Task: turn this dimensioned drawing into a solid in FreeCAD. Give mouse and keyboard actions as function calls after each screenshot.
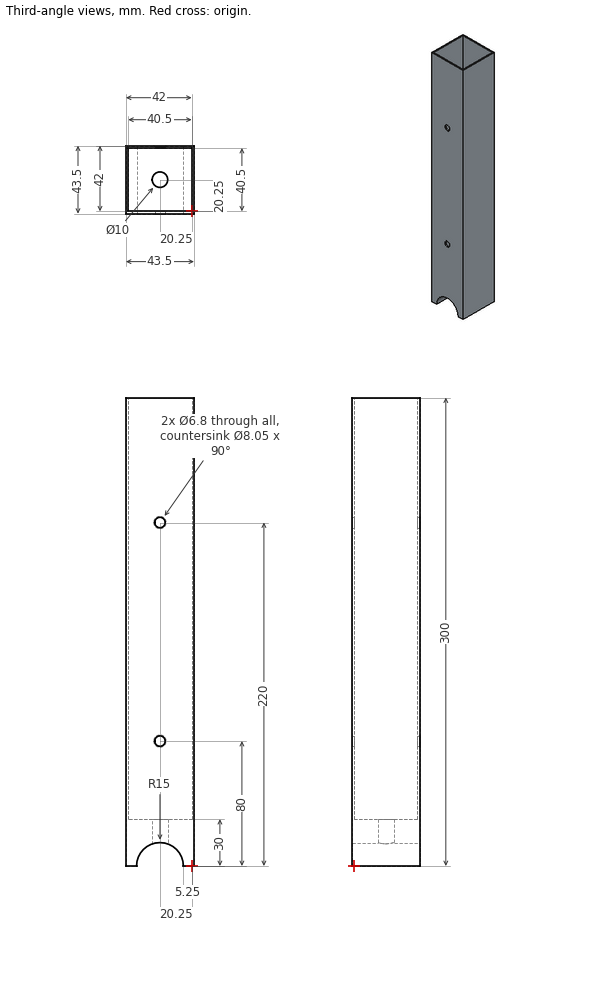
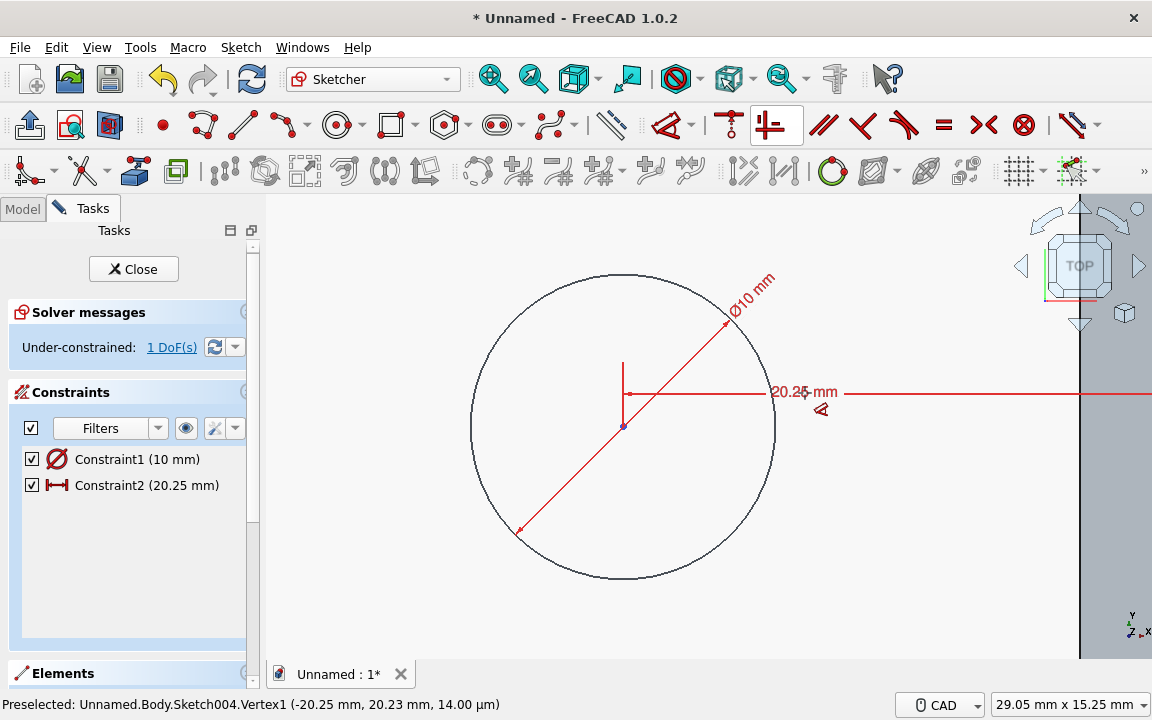
click(623, 427)
click(589, 529)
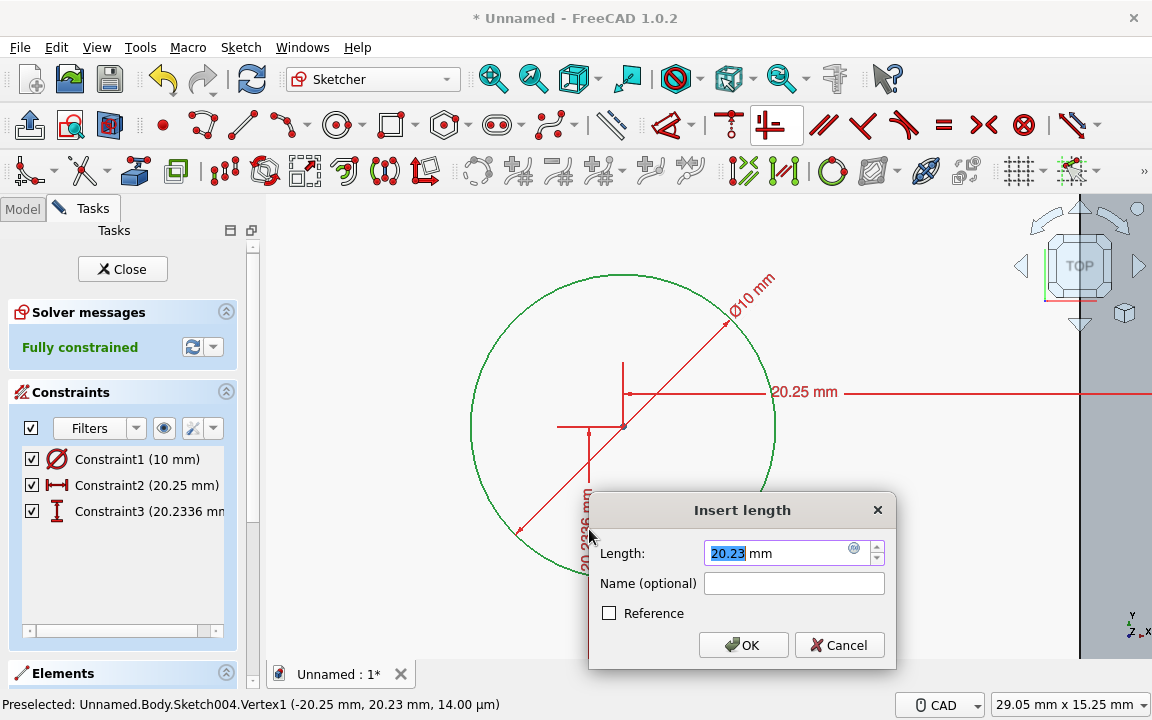
text(20.25)
key(Return)
key(Escape)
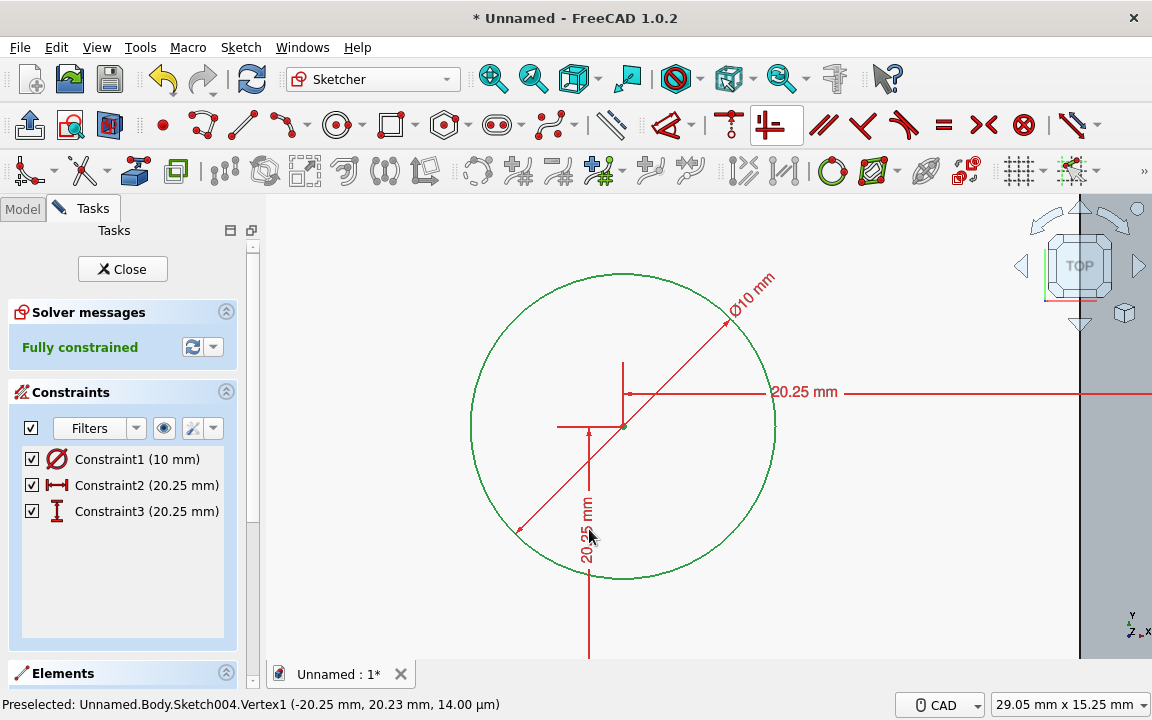
click(123, 269)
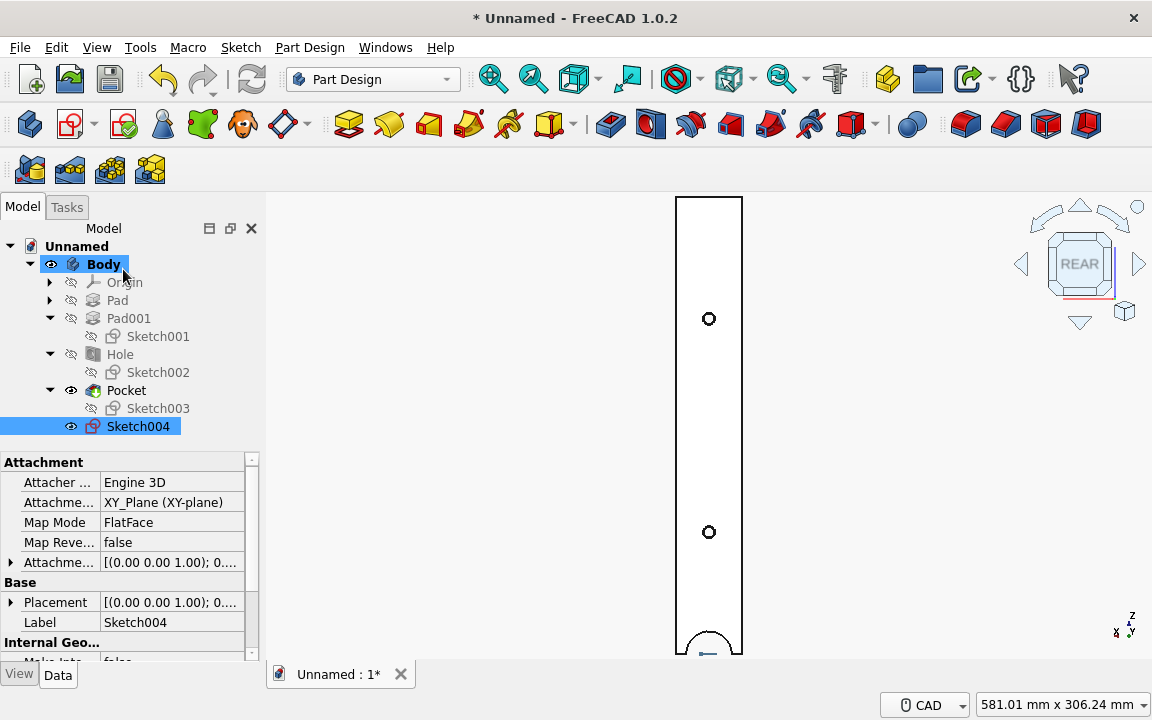
click(612, 124)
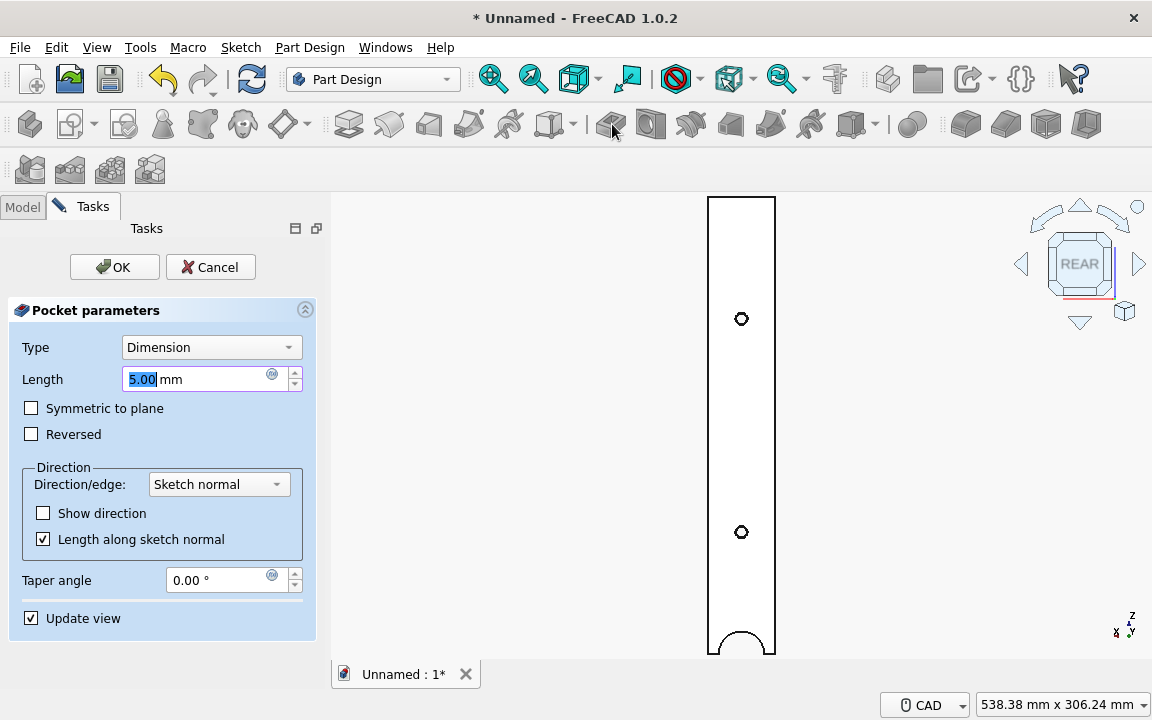
click(212, 348)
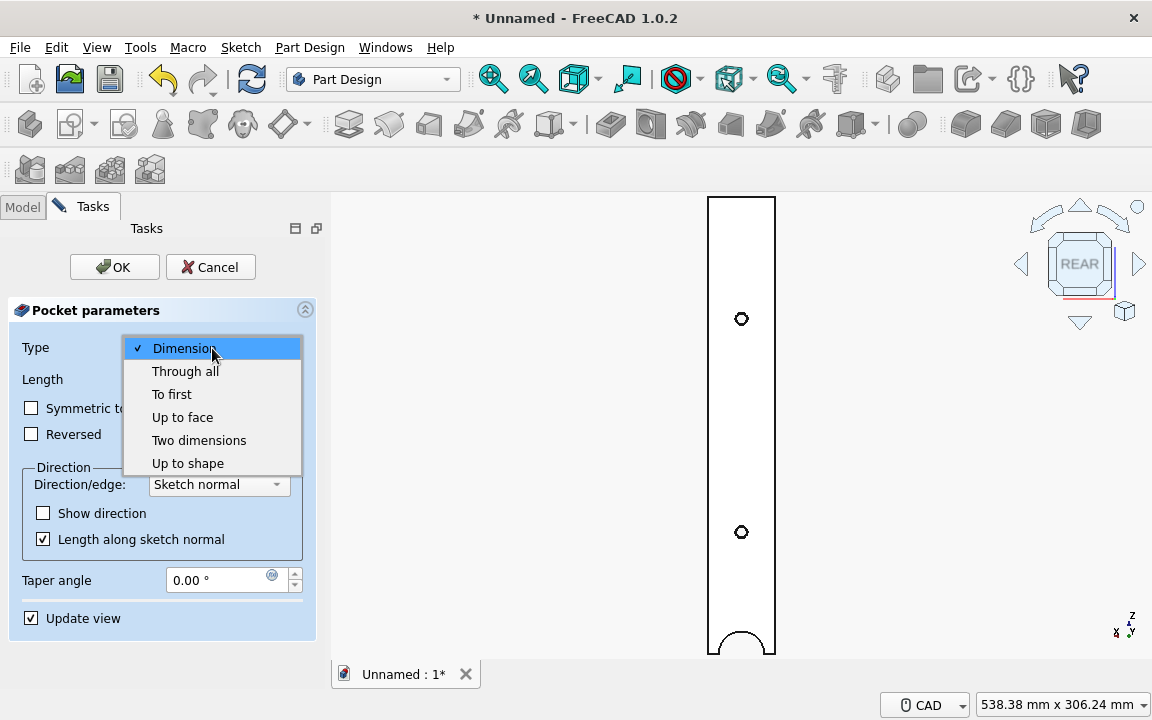
click(212, 372)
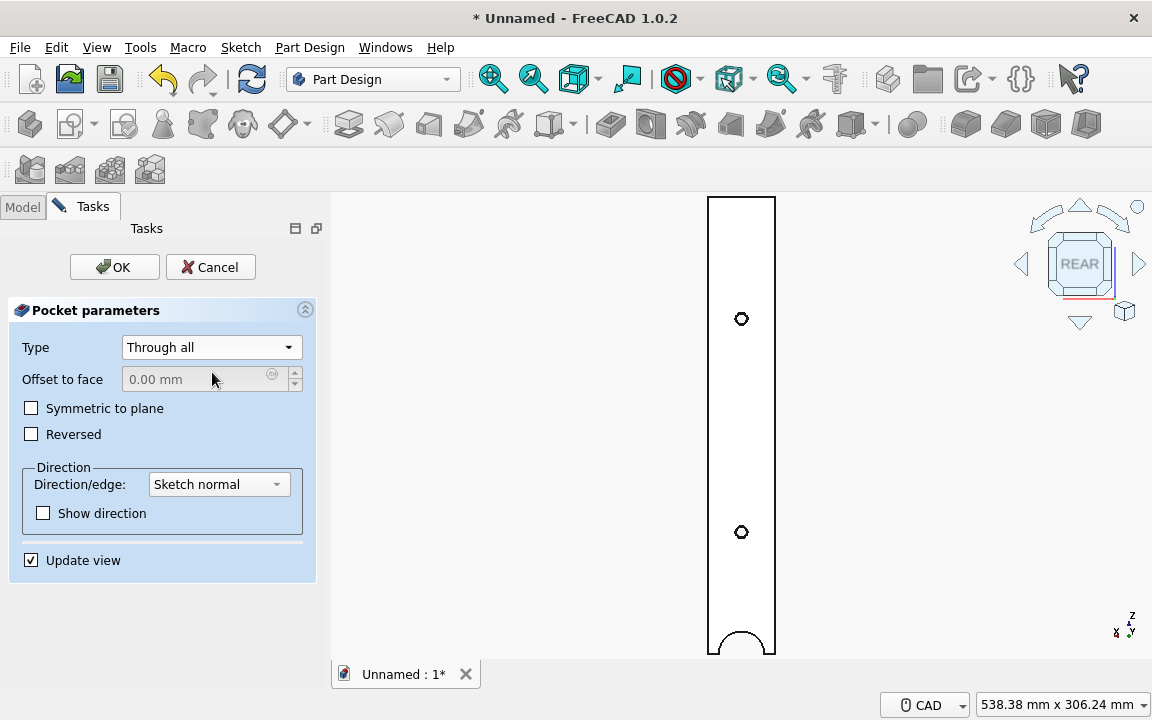
click(30, 434)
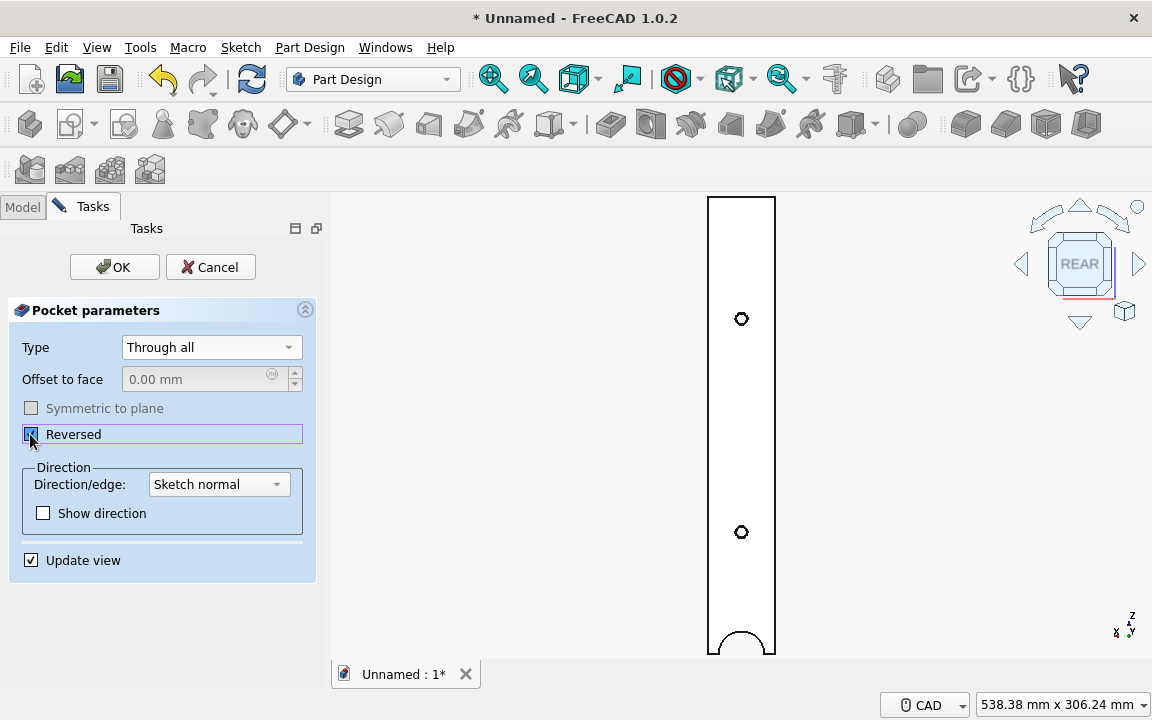
click(115, 267)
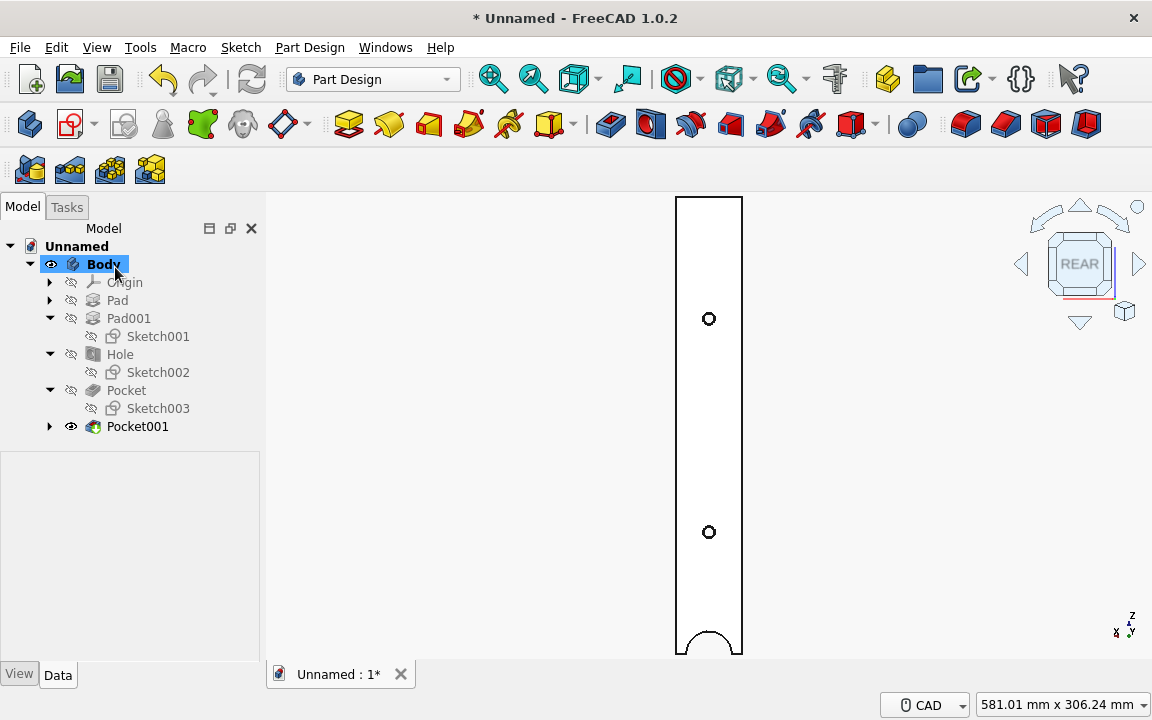
key(0)